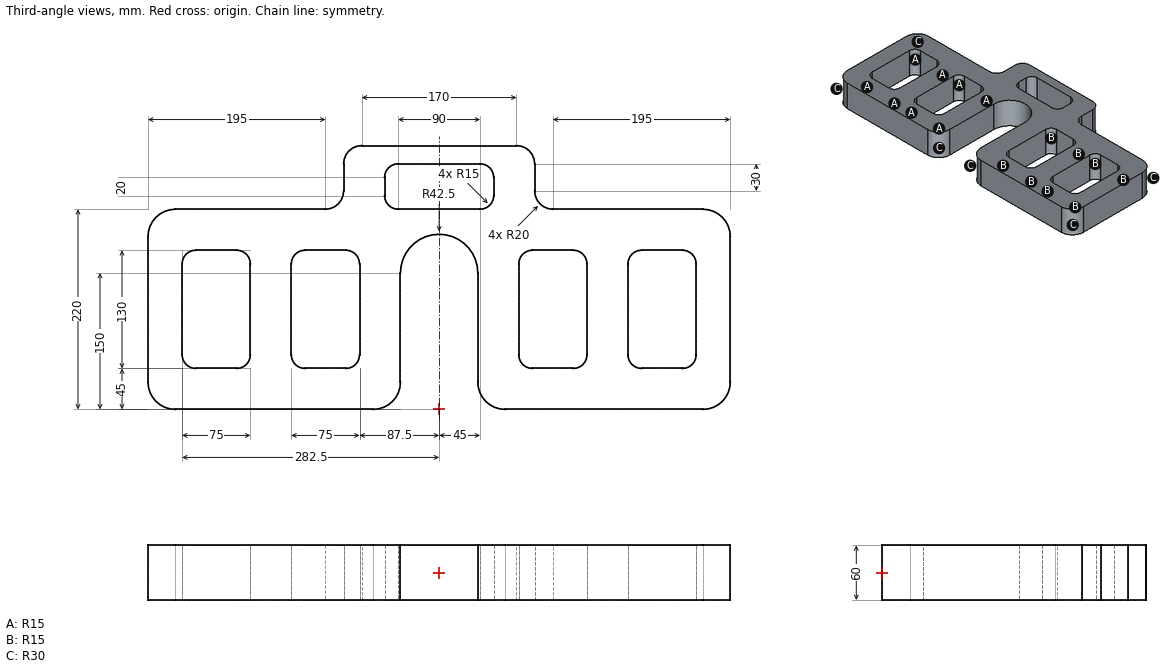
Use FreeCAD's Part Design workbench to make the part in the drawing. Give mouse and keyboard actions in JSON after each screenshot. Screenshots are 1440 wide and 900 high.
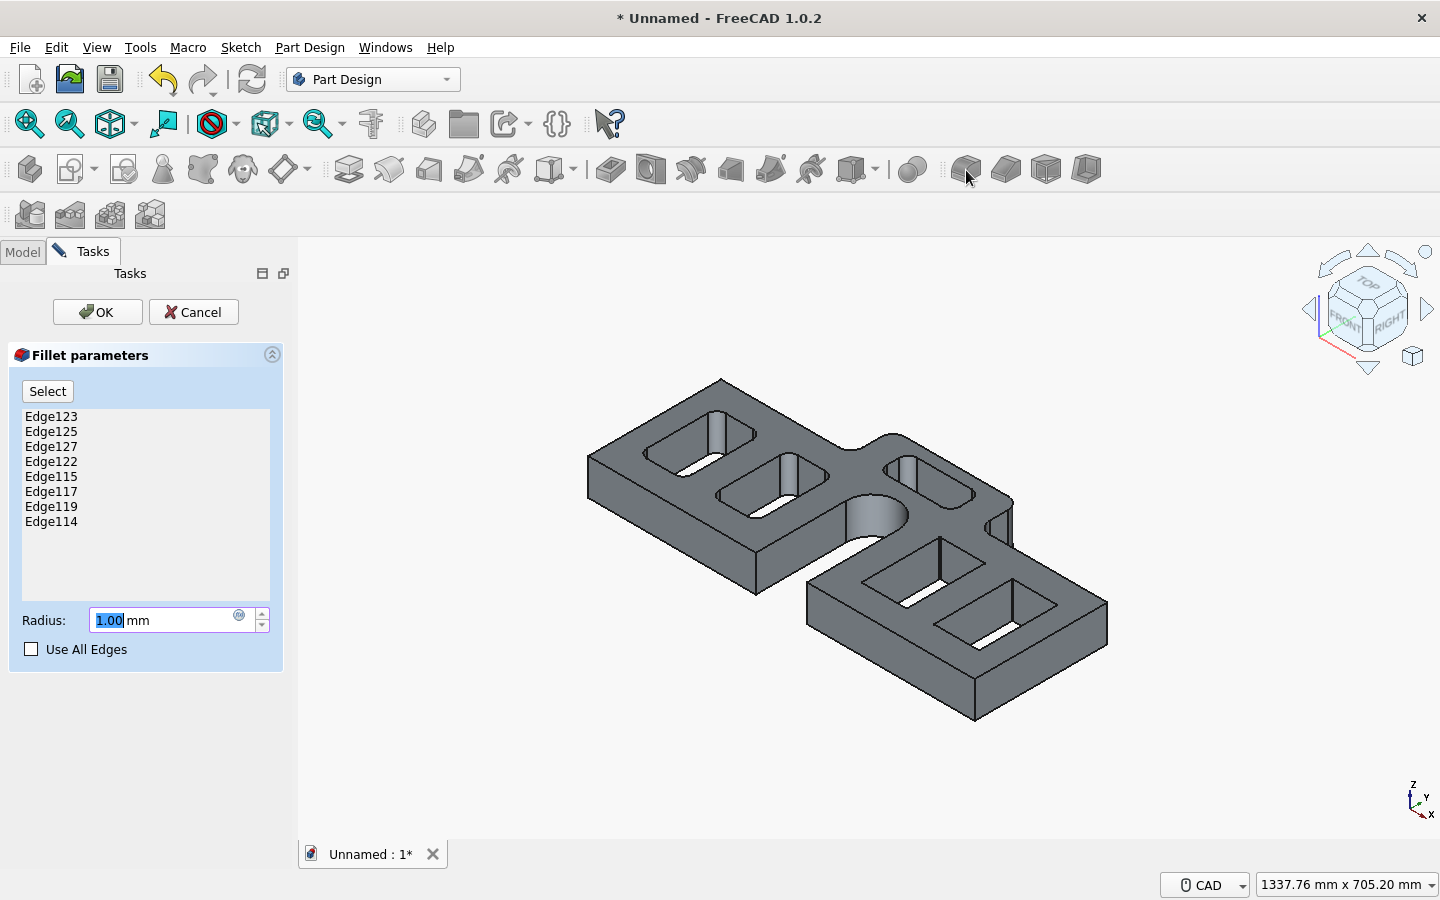
{"action": "type", "text": "15"}
{"action": "key", "text": "Tab"}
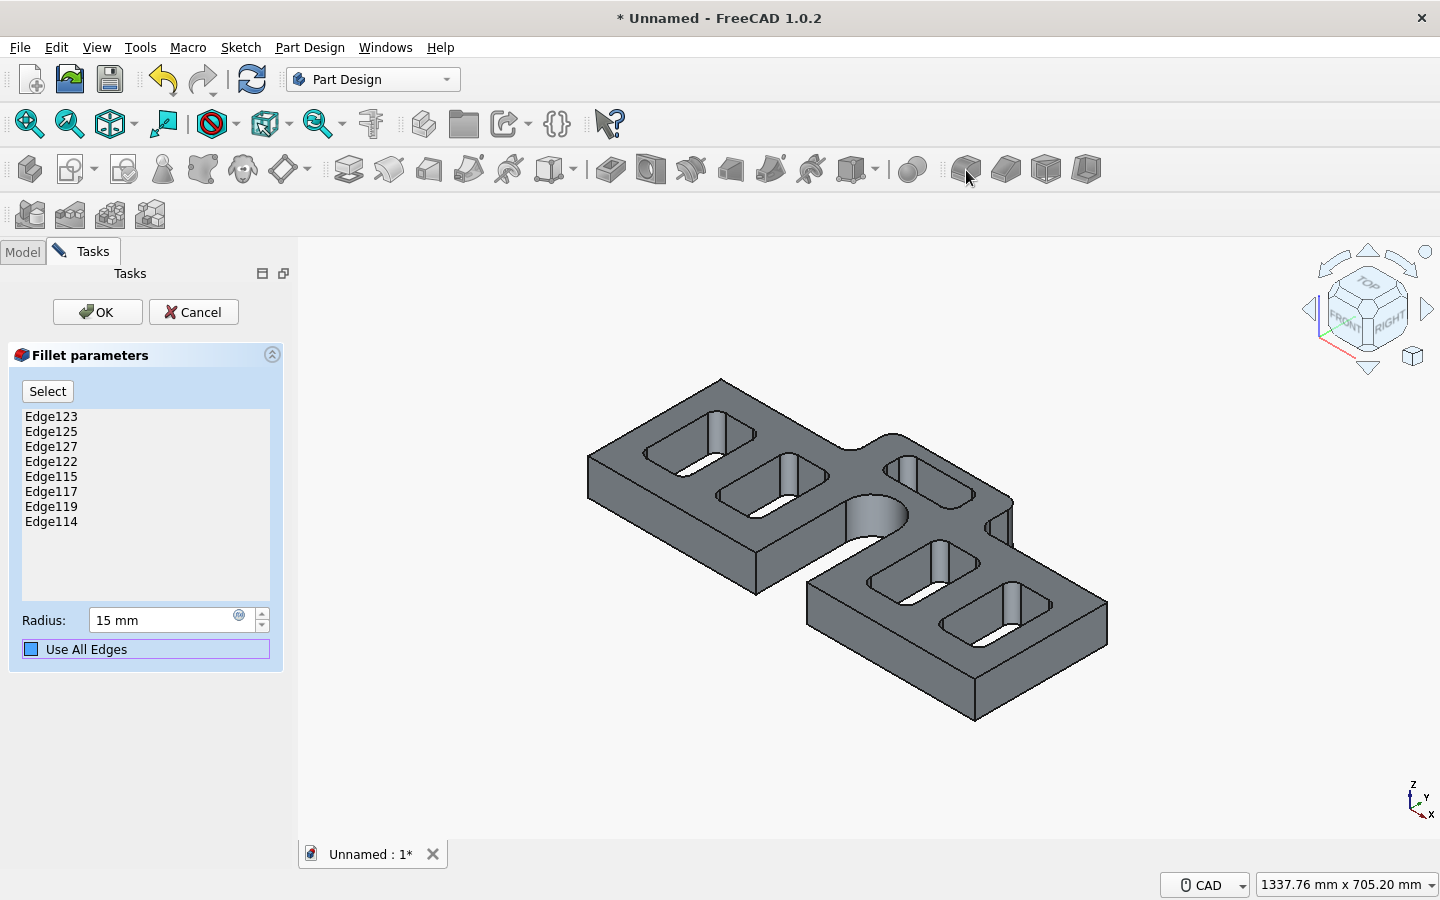
{"action": "left_click", "coordinate": [98, 312]}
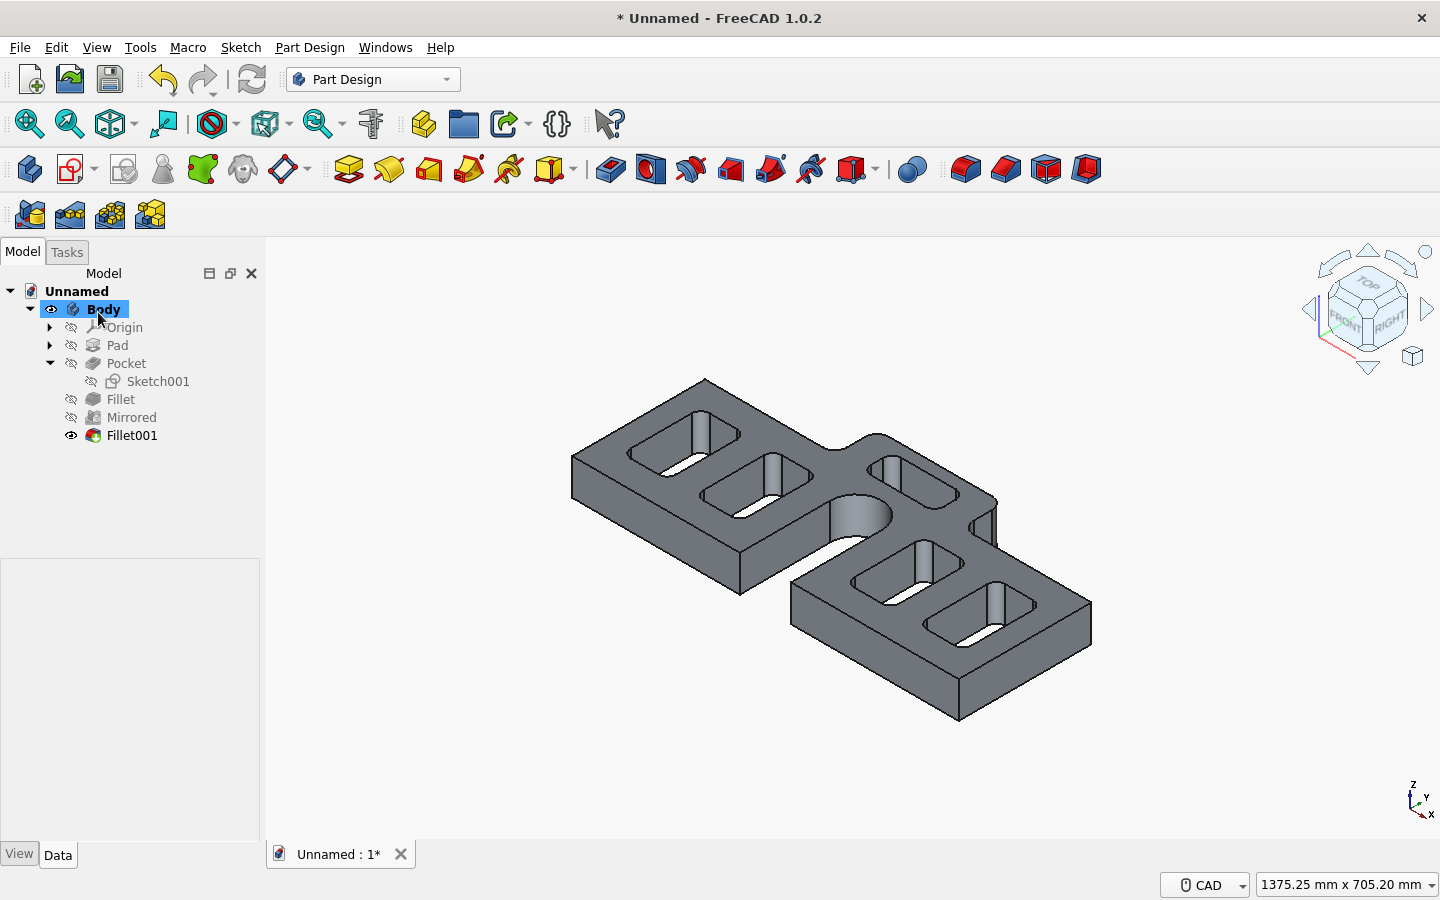
{"action": "left_click", "coordinate": [740, 573]}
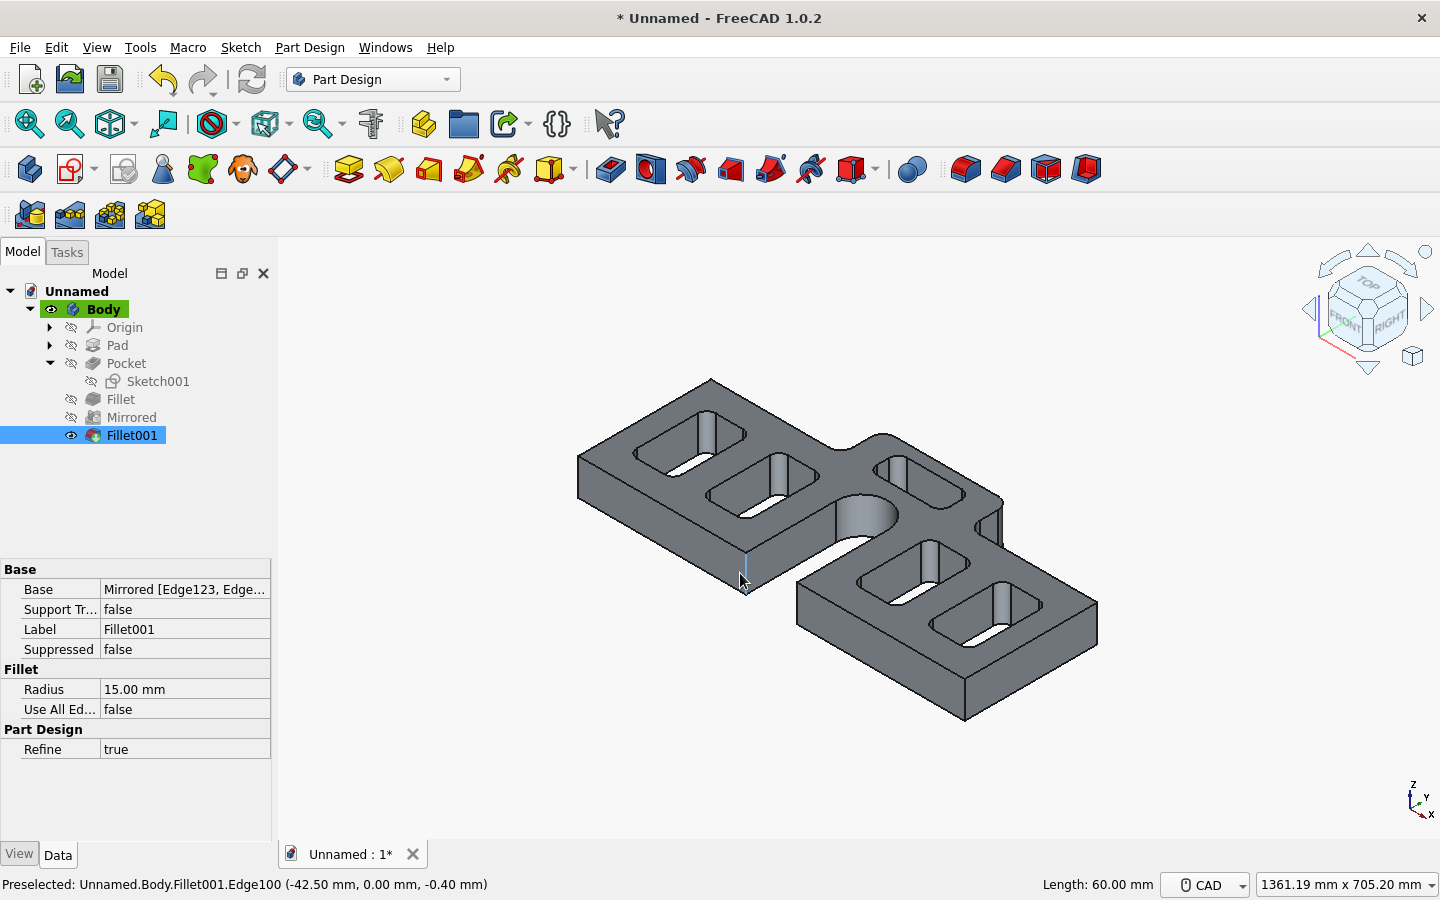
{"action": "left_click", "coordinate": [965, 699], "text": "ctrl"}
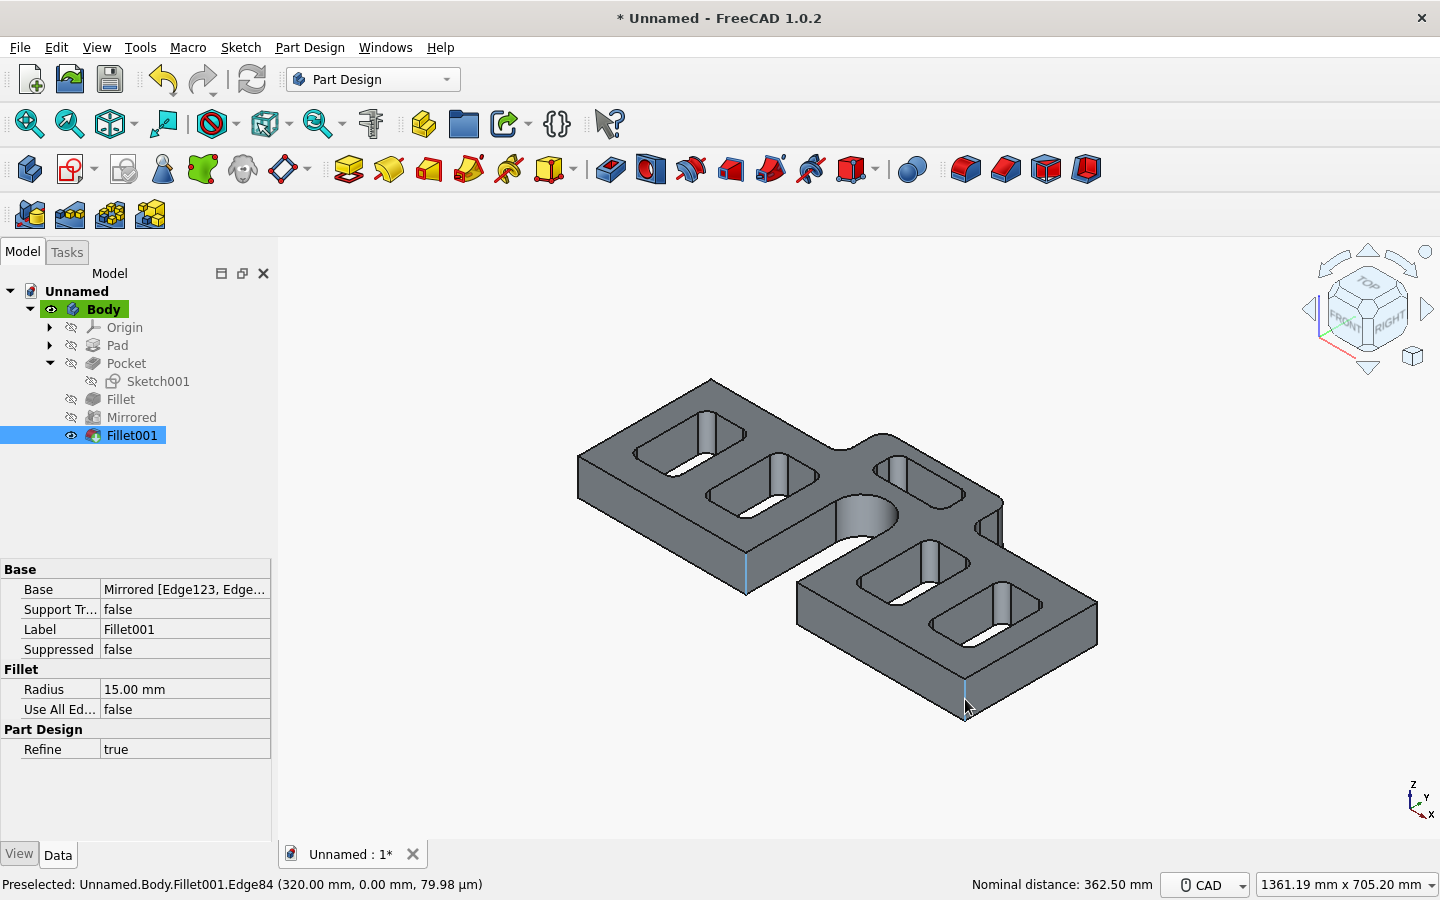
{"action": "key", "text": "2"}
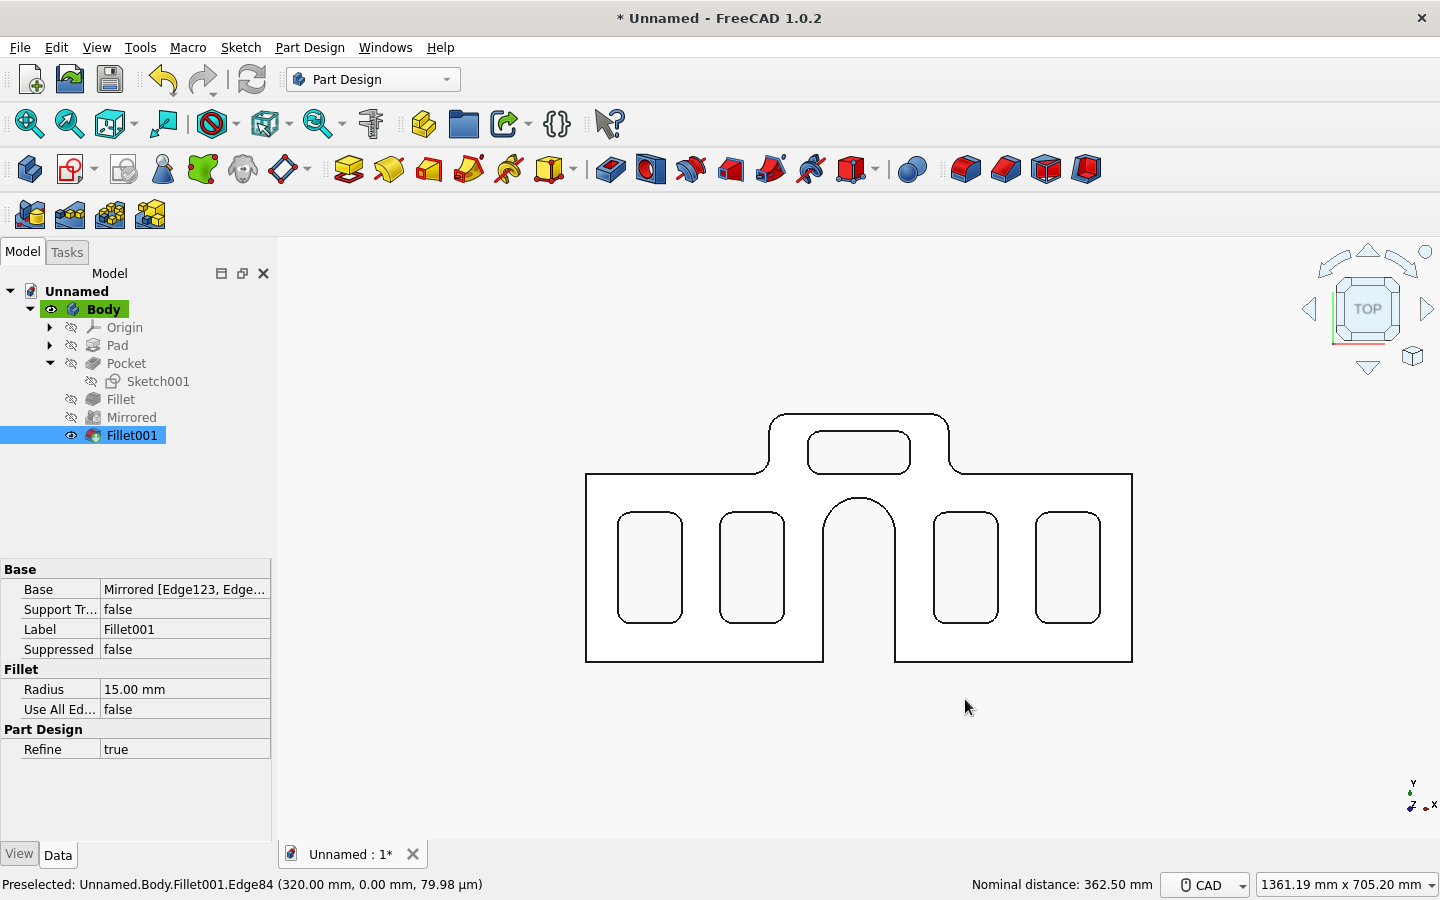
{"action": "key", "text": "0"}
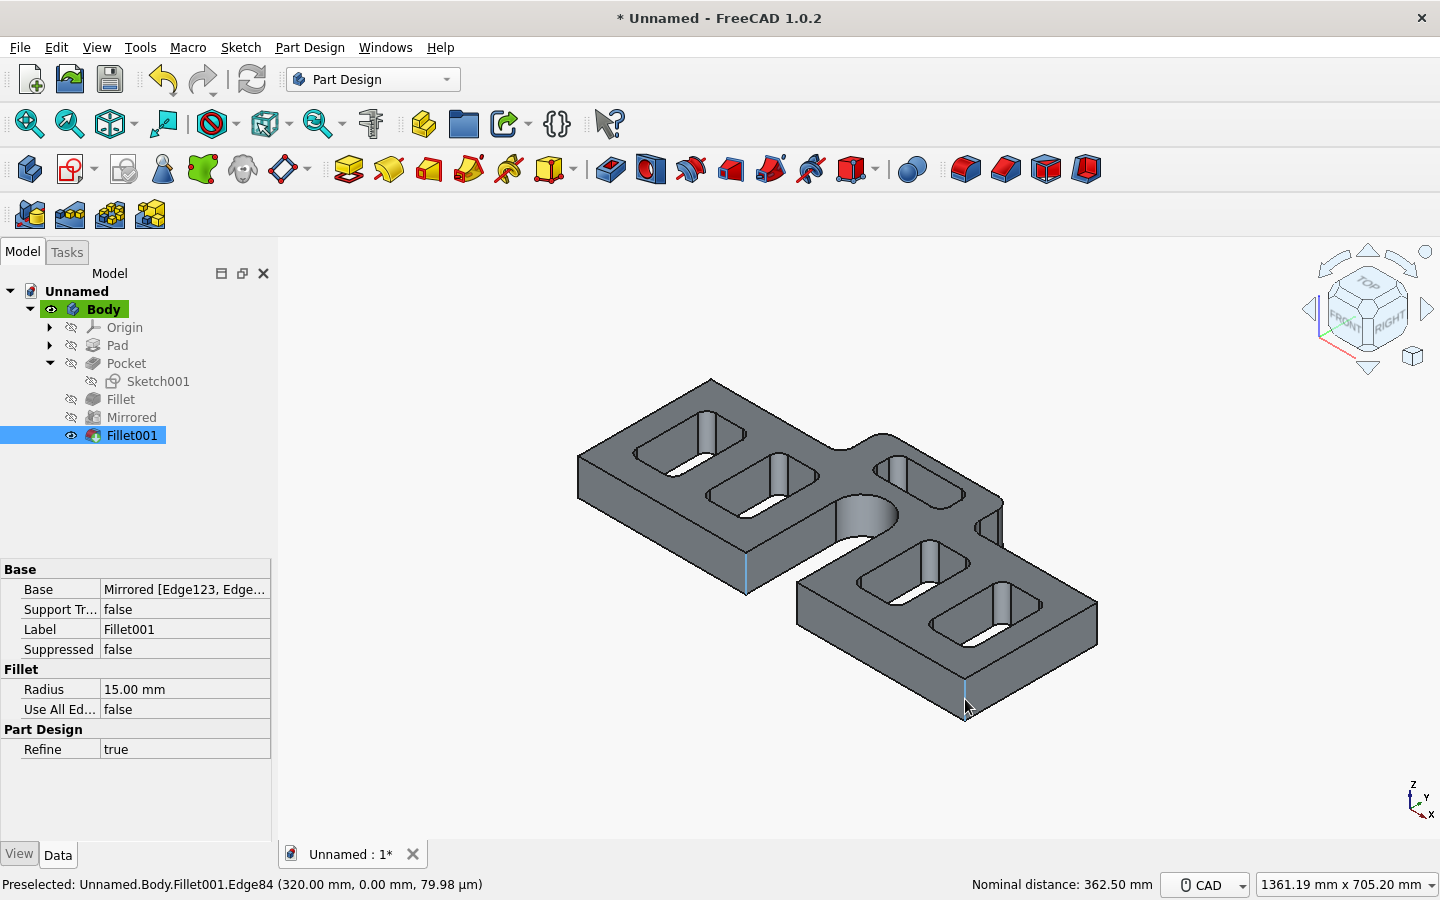
{"action": "key", "text": "1"}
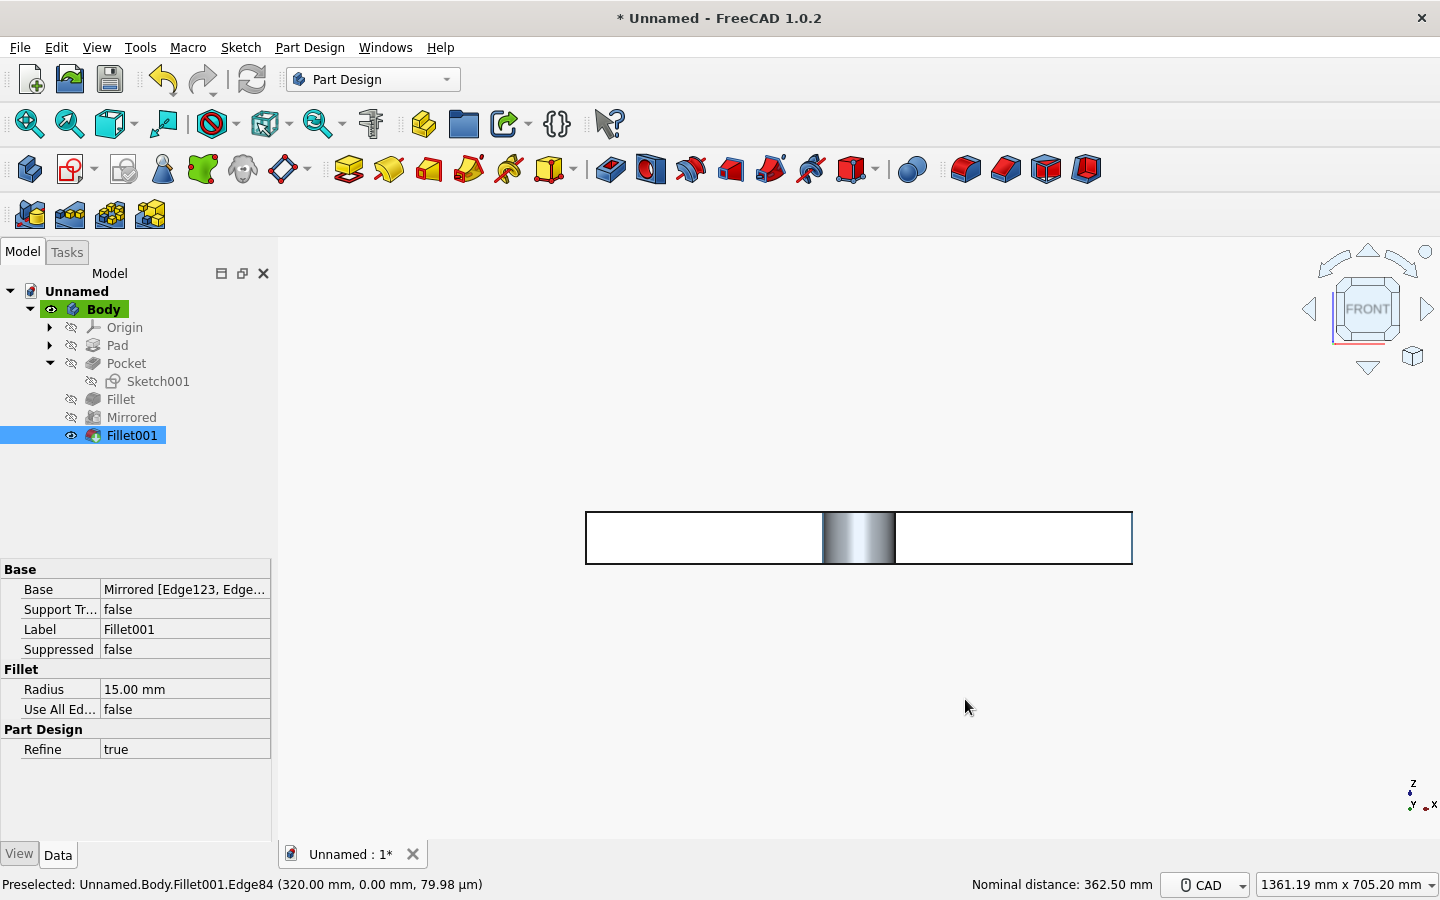
{"action": "left_click", "coordinate": [586, 537], "text": "ctrl"}